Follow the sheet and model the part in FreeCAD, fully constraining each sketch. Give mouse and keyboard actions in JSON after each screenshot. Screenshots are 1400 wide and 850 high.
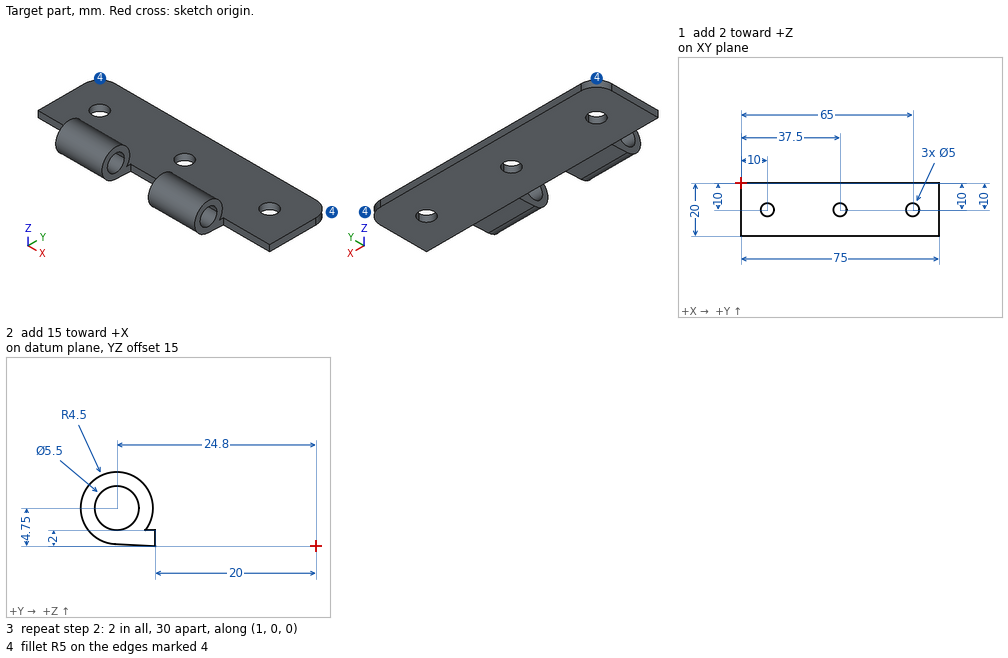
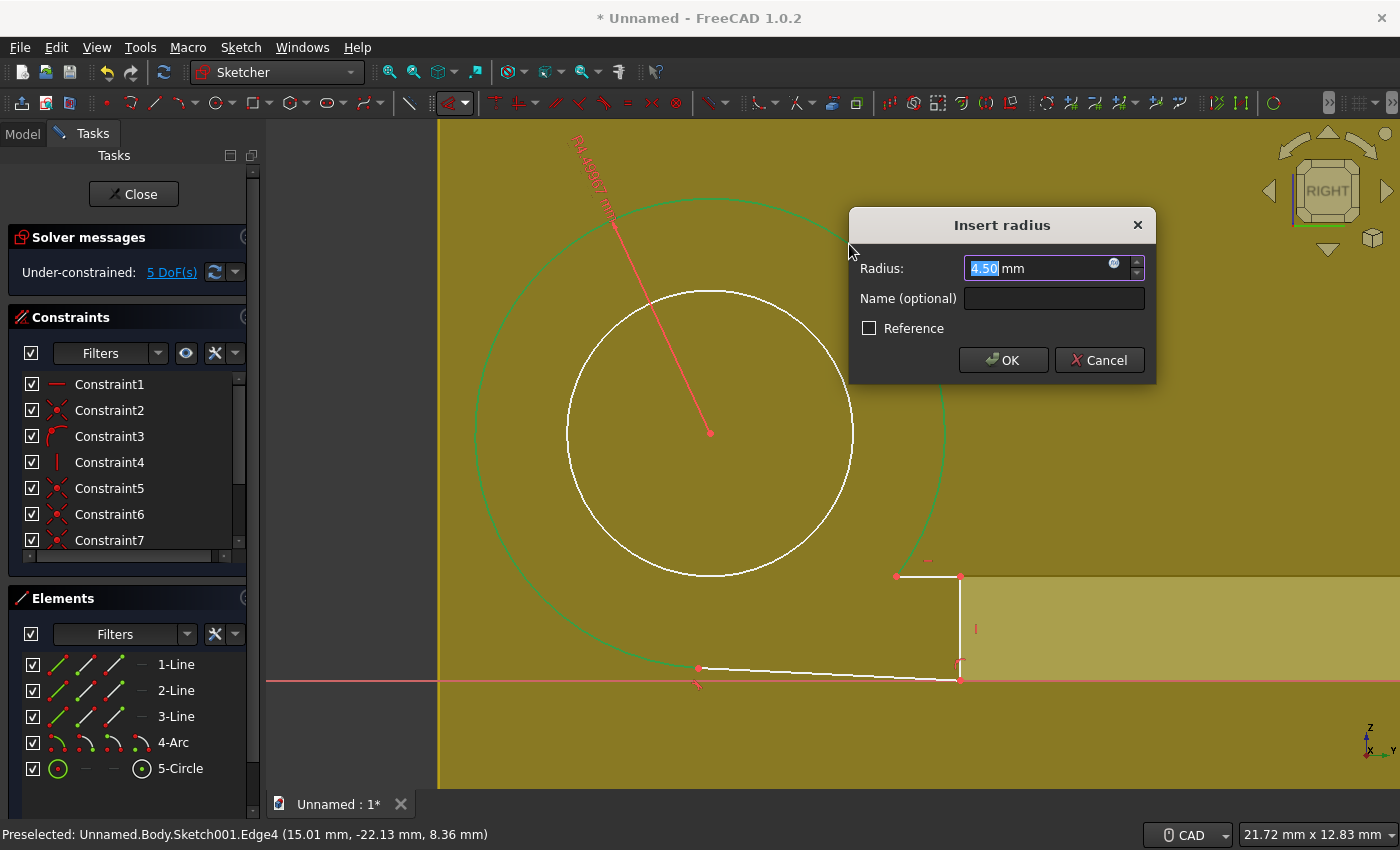
{"action": "type", "text": "4.5"}
{"action": "key", "text": "Return"}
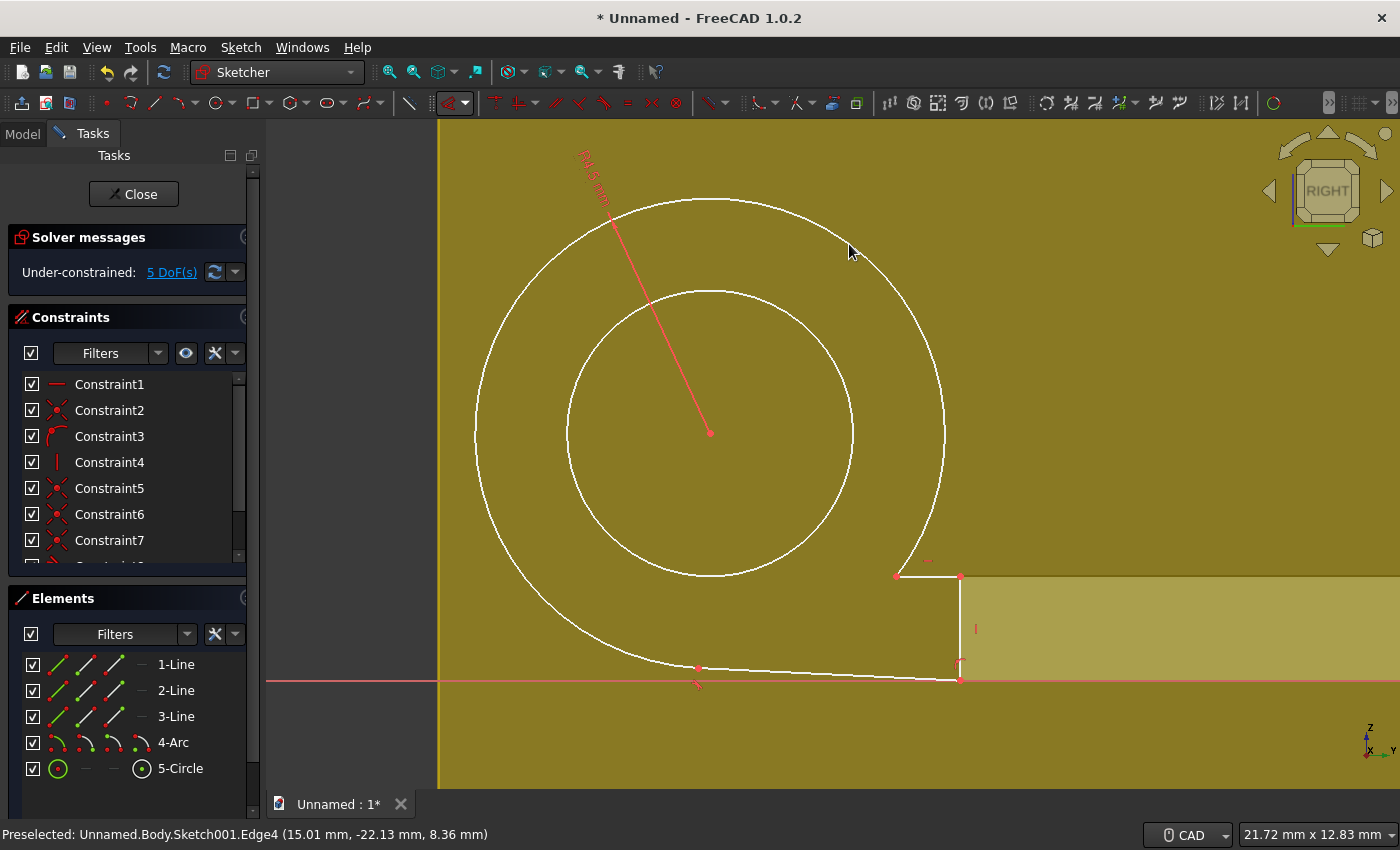
{"action": "left_click", "coordinate": [811, 332]}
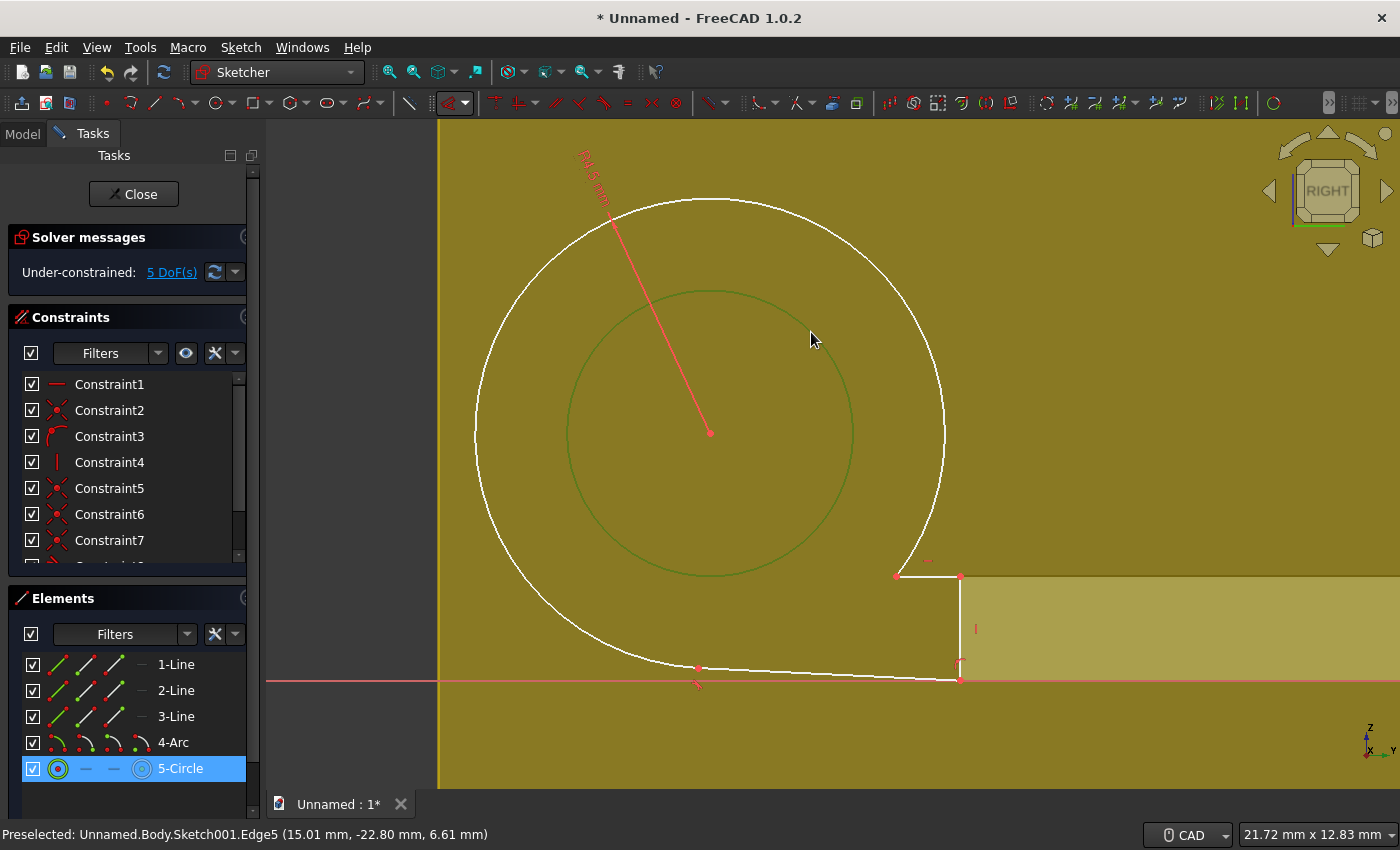
{"action": "key", "text": "k o"}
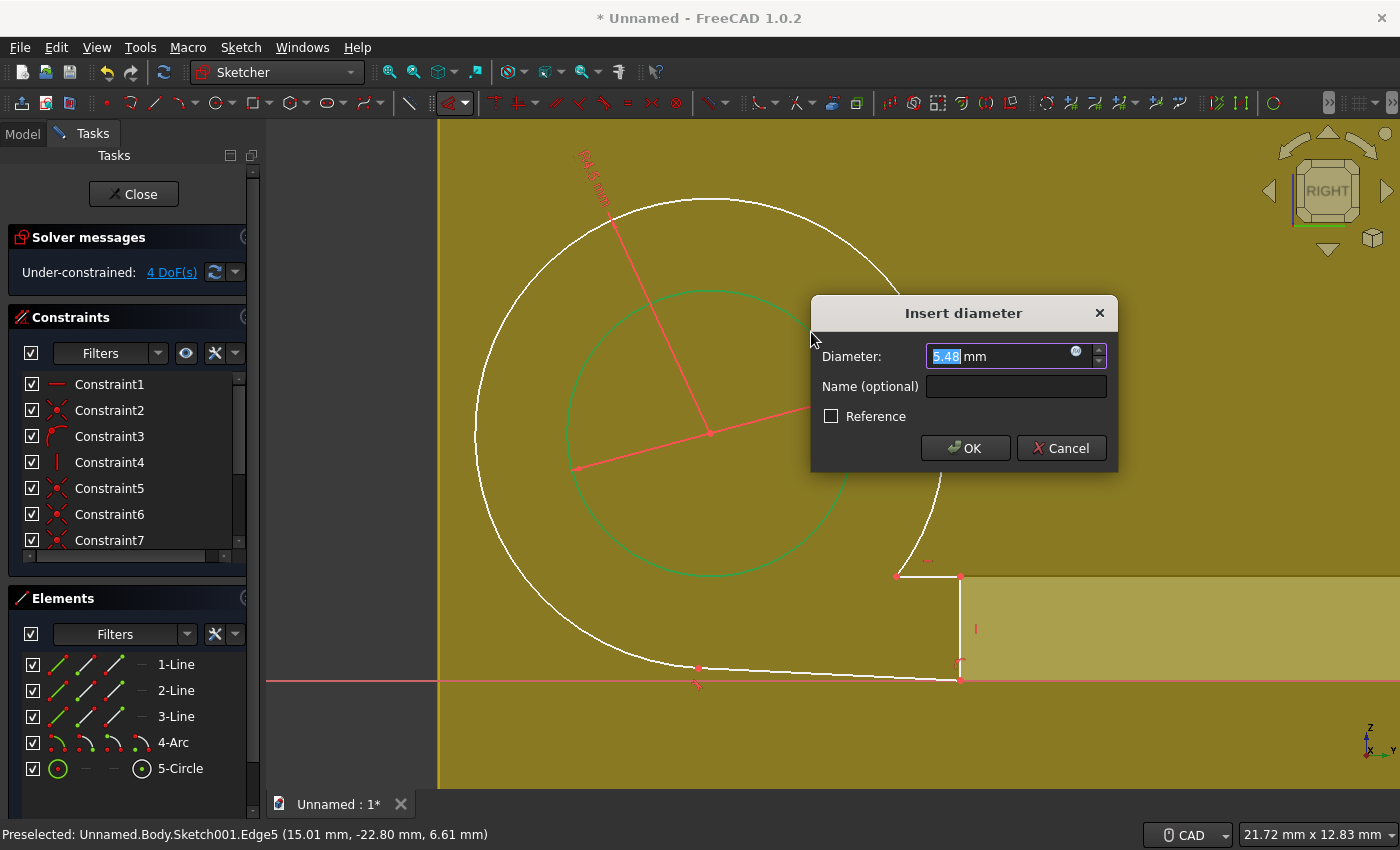
{"action": "type", "text": "5.5"}
{"action": "key", "text": "Return"}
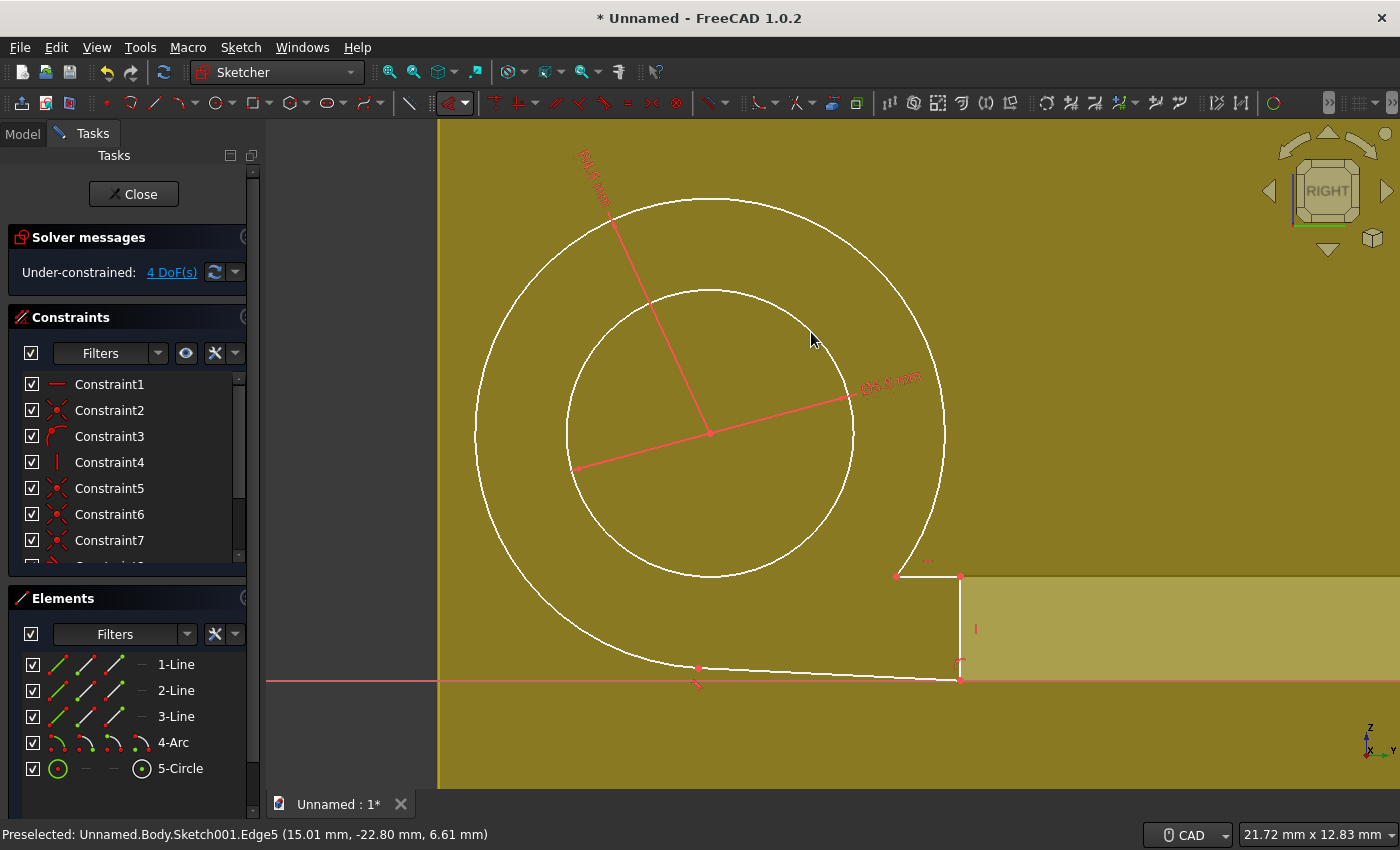
{"action": "left_click", "coordinate": [960, 608]}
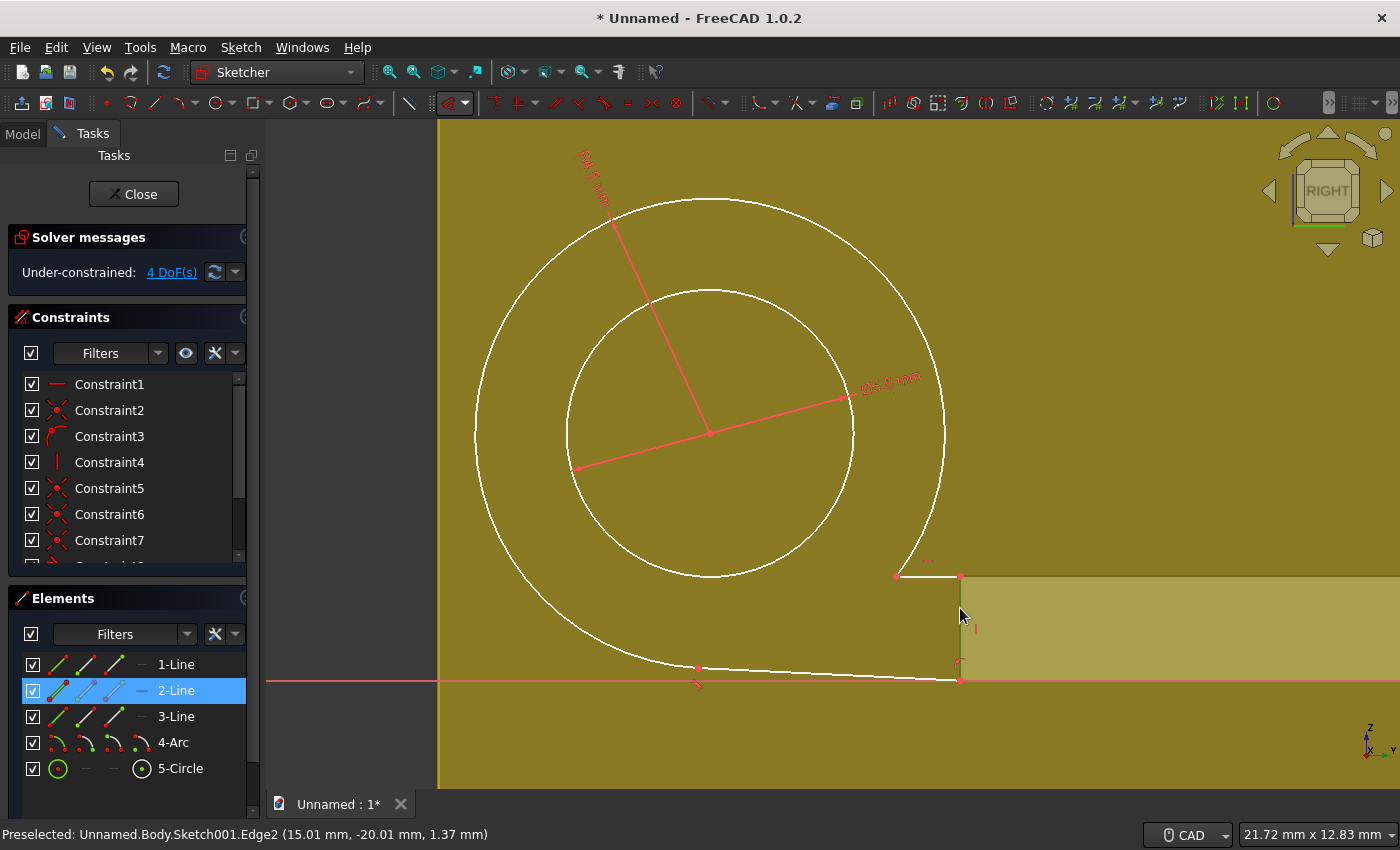
{"action": "key", "text": "i"}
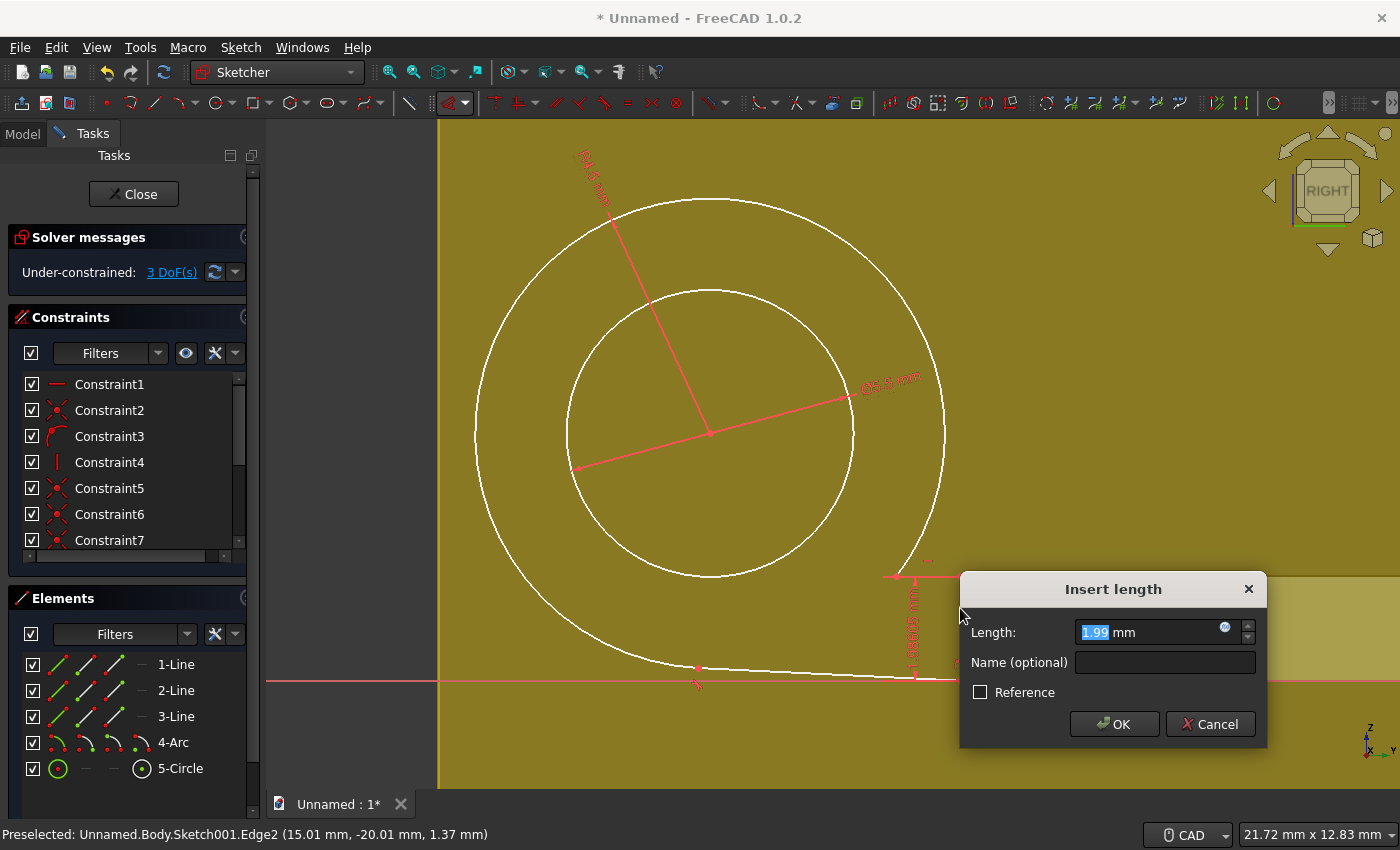
{"action": "type", "text": "2"}
{"action": "key", "text": "Return"}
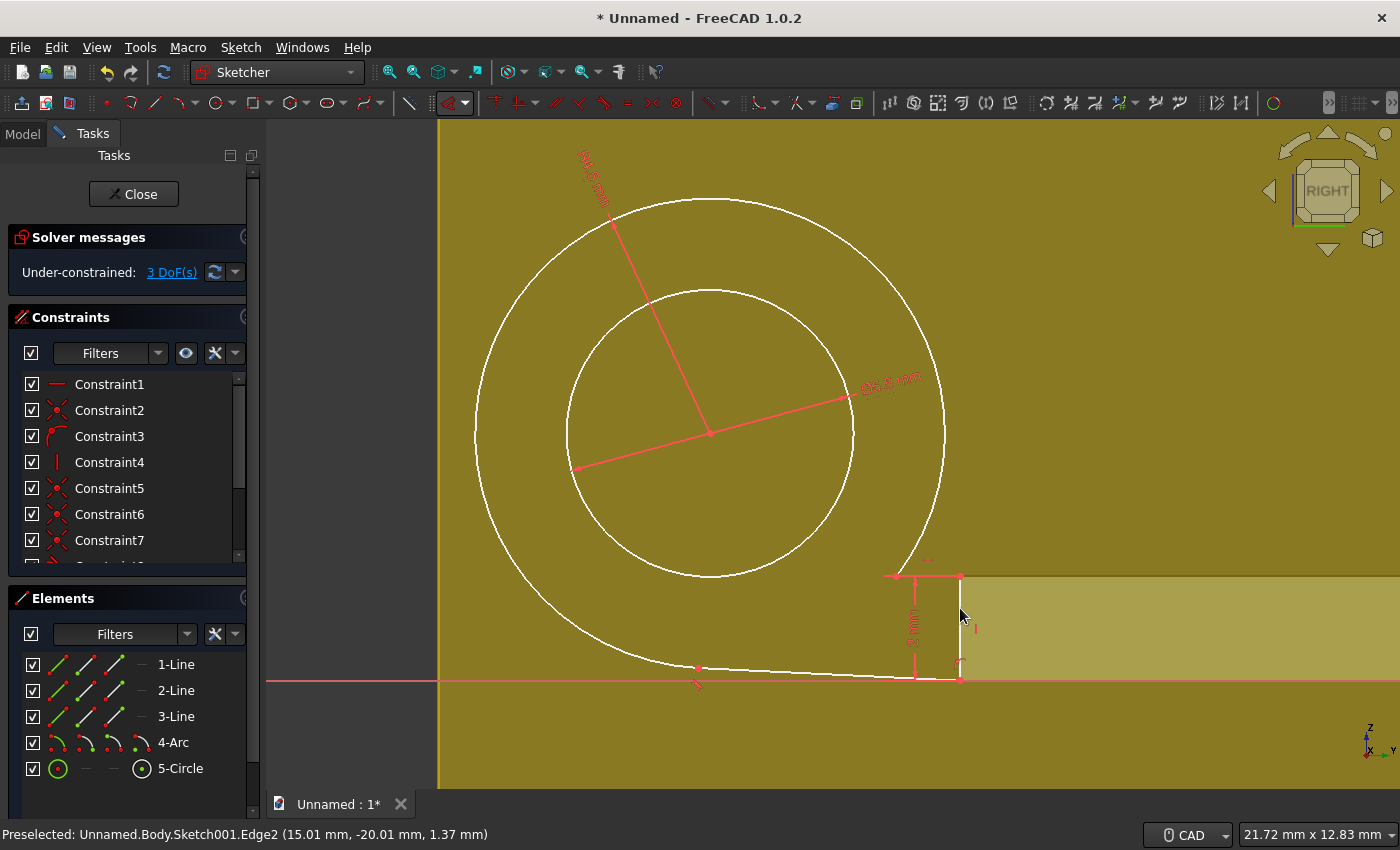
{"action": "left_click", "coordinate": [960, 576]}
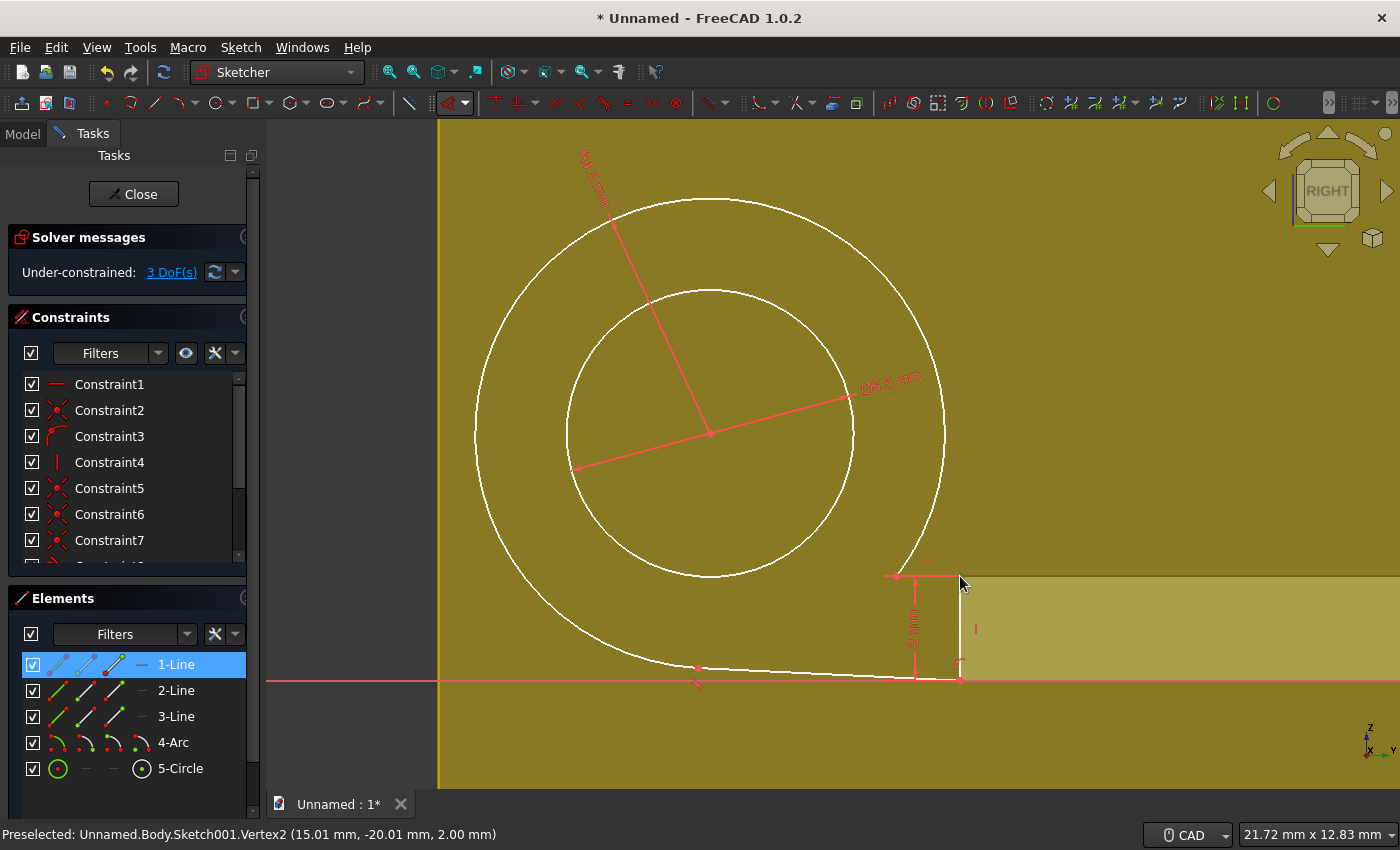
{"action": "key", "text": "l"}